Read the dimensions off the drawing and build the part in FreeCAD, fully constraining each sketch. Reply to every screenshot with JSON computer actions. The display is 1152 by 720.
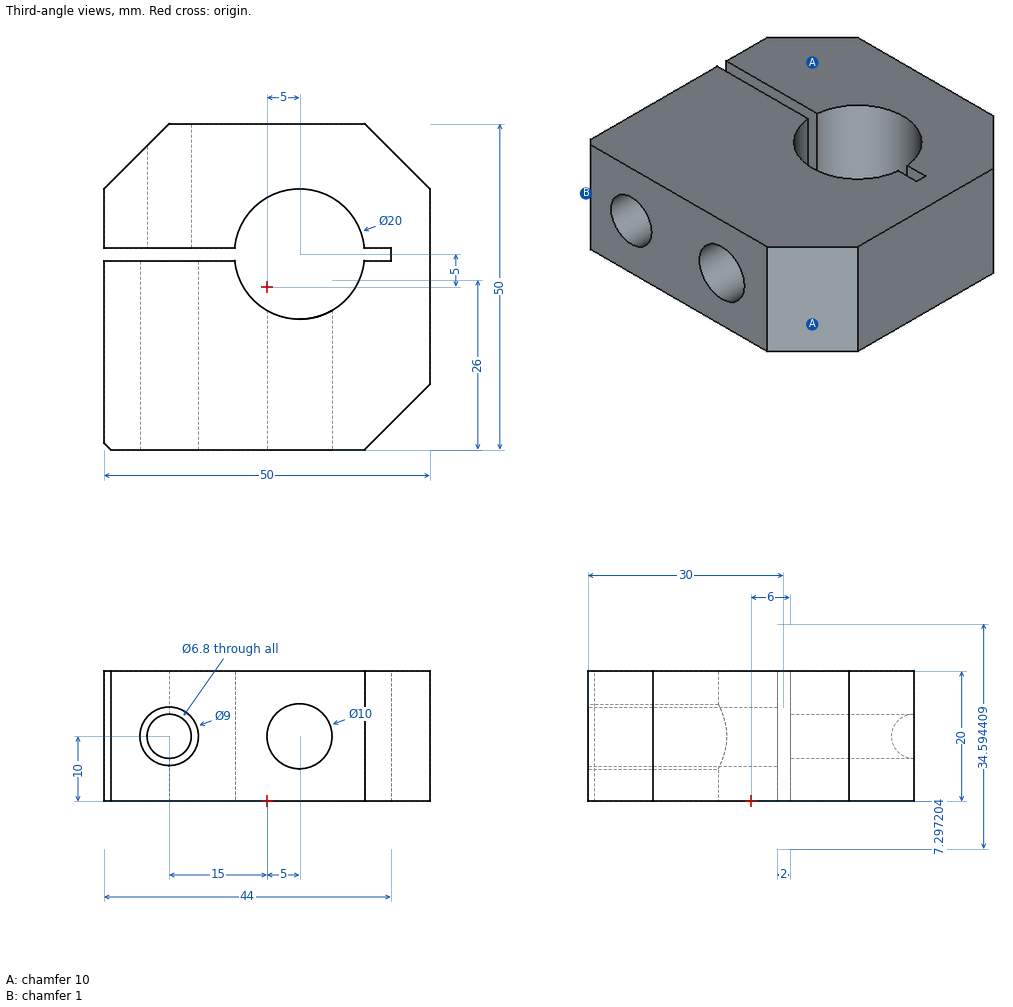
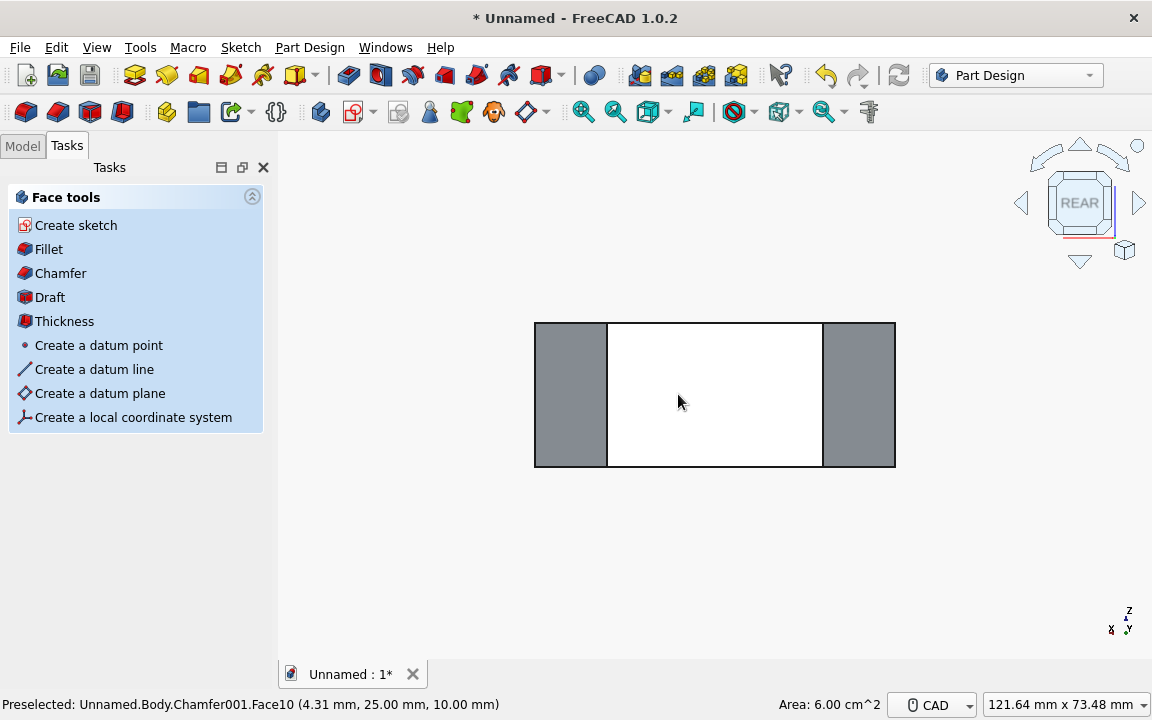
{"action": "left_click", "coordinate": [354, 112]}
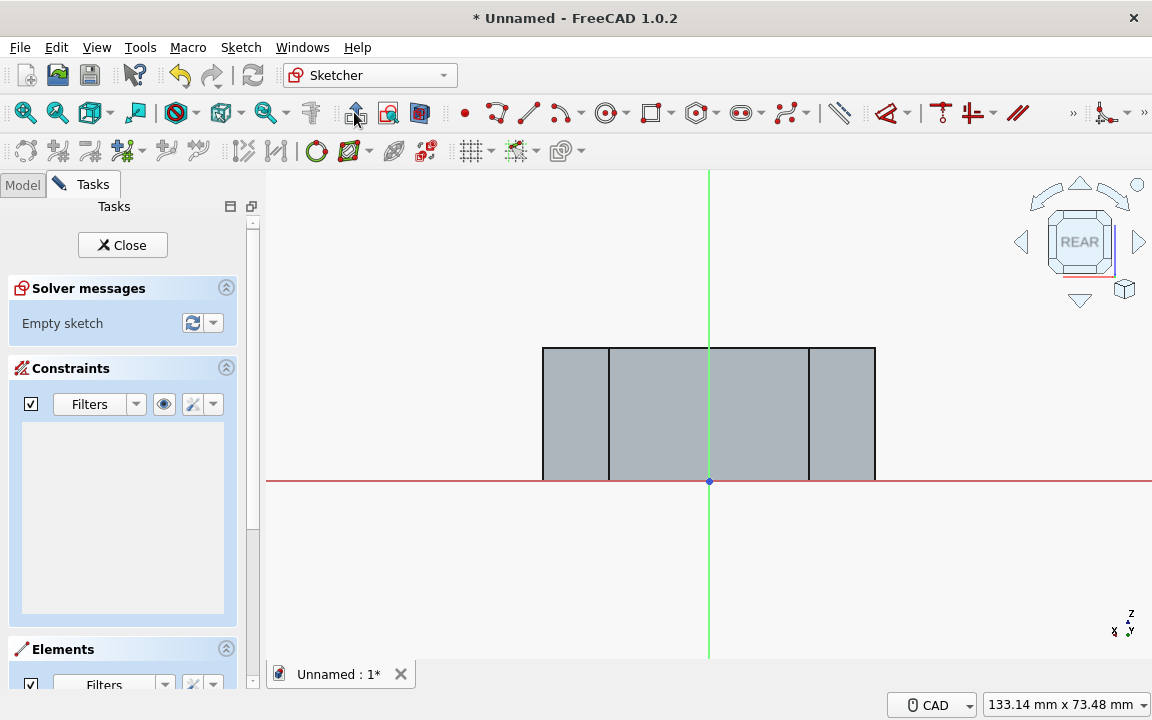
{"action": "scroll", "coordinate": [835, 414], "scroll_direction": "up", "scroll_amount": 10}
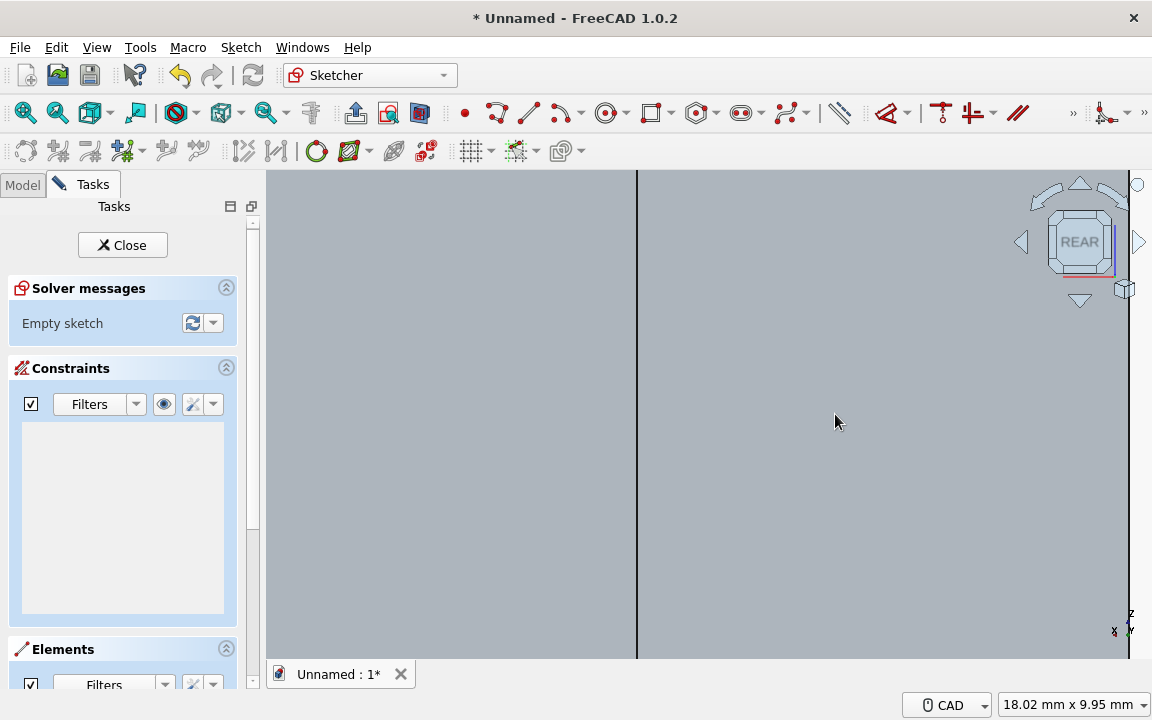
{"action": "left_click", "coordinate": [606, 114]}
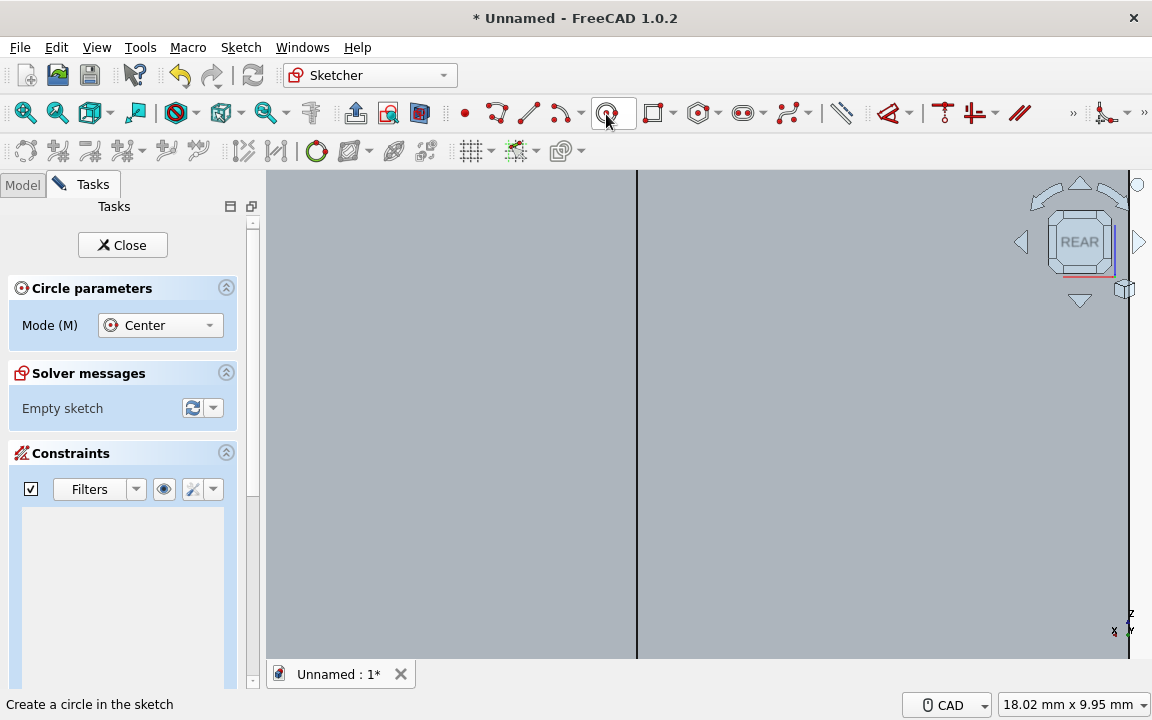
{"action": "left_click", "coordinate": [637, 415]}
{"action": "mouse_move", "coordinate": [756, 296]}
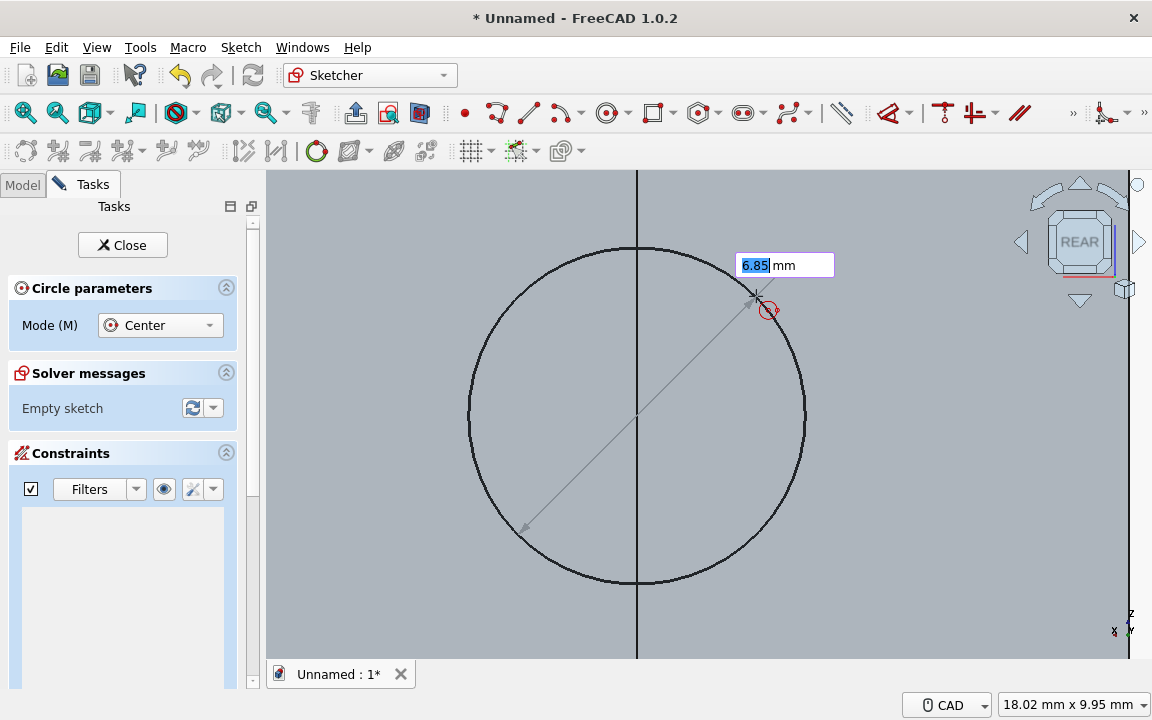
{"action": "type", "text": "6.8"}
{"action": "key", "text": "Return"}
{"action": "key", "text": "Escape"}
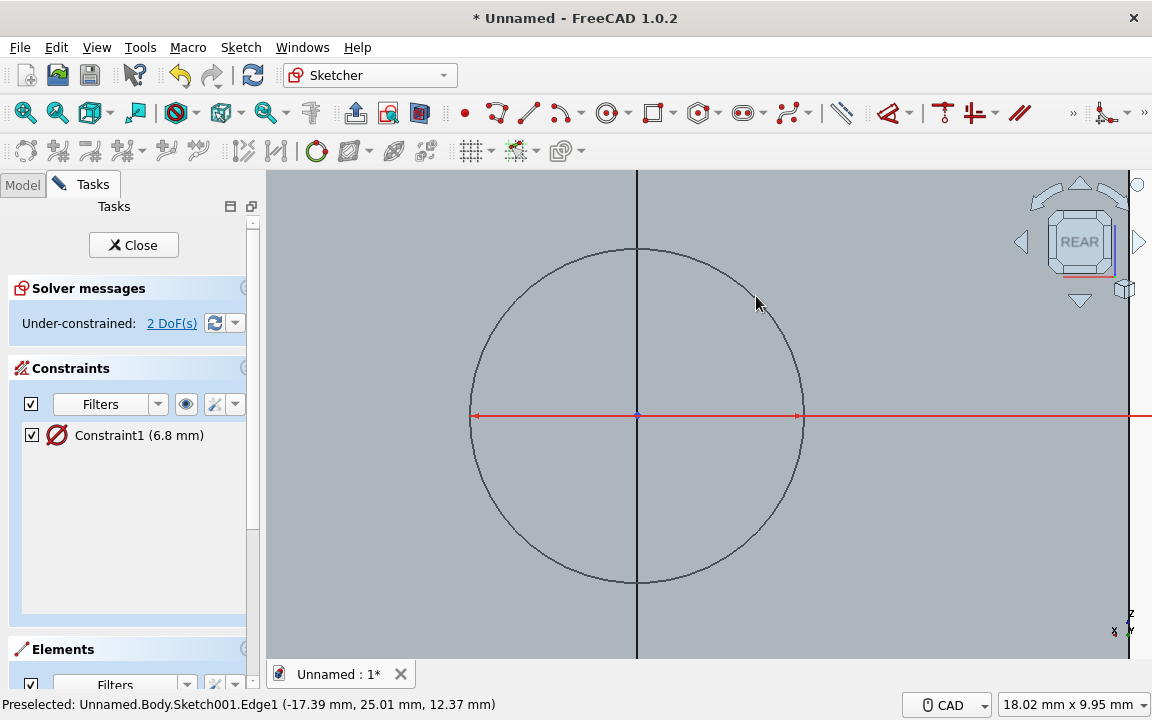
{"action": "left_click", "coordinate": [888, 114]}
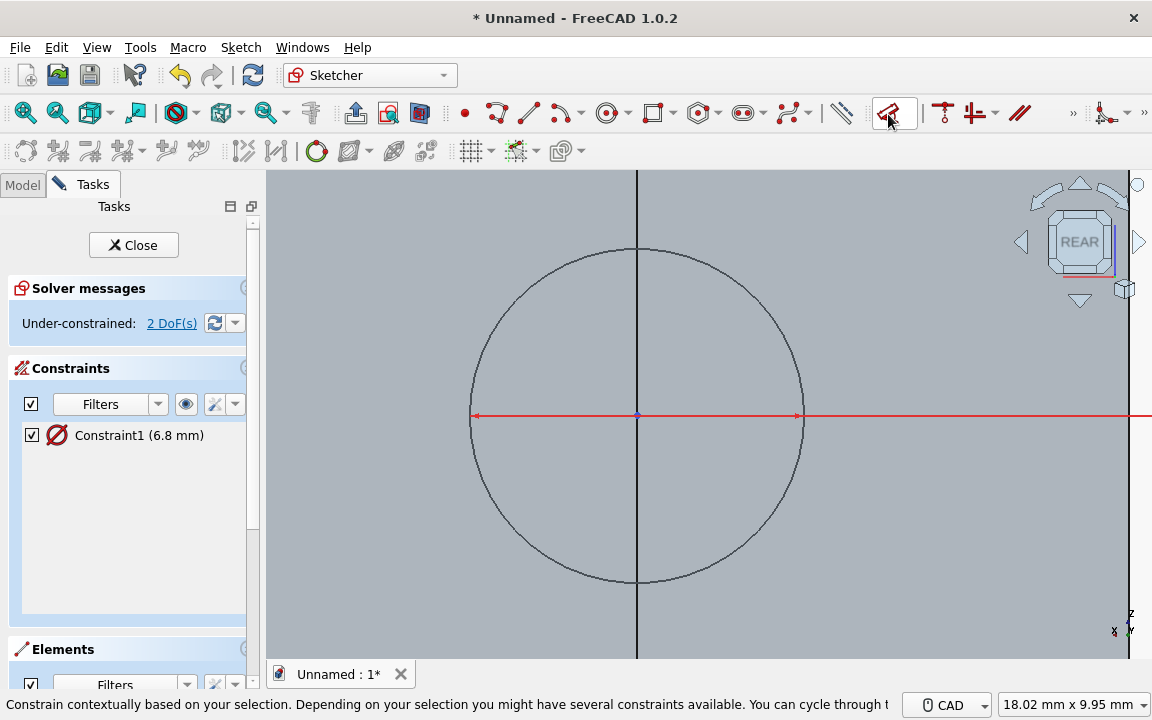
{"action": "left_click", "coordinate": [637, 416]}
{"action": "left_click", "coordinate": [387, 382]}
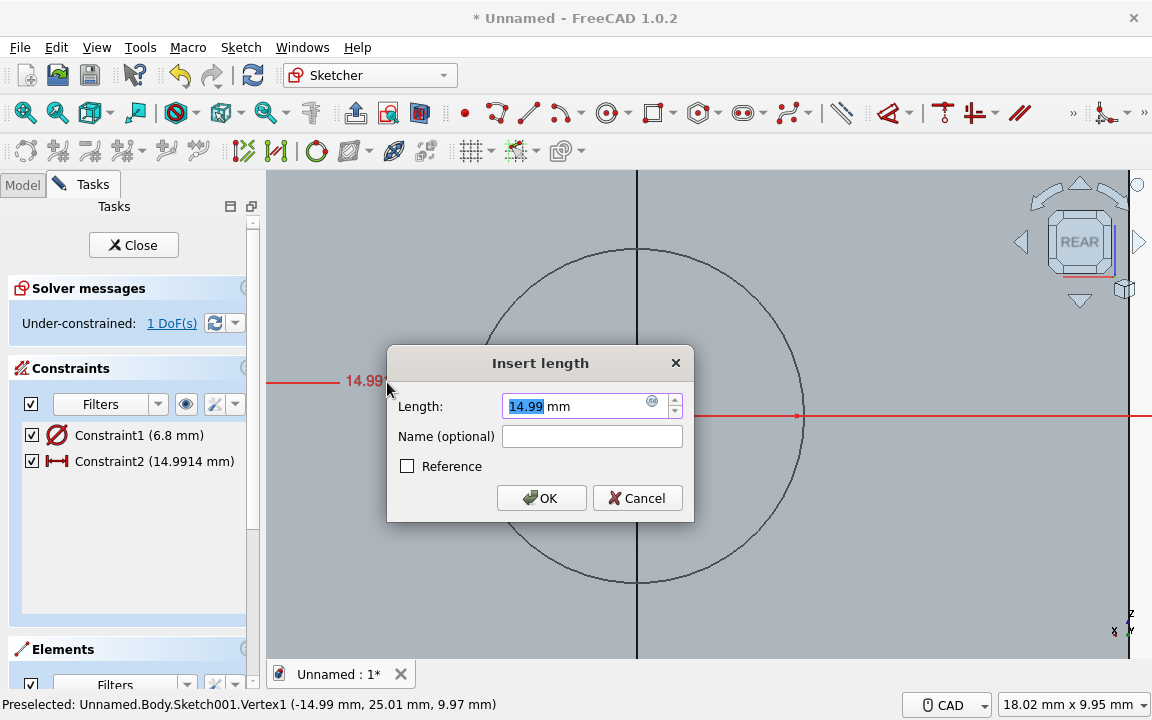
{"action": "type", "text": "15"}
{"action": "key", "text": "Return"}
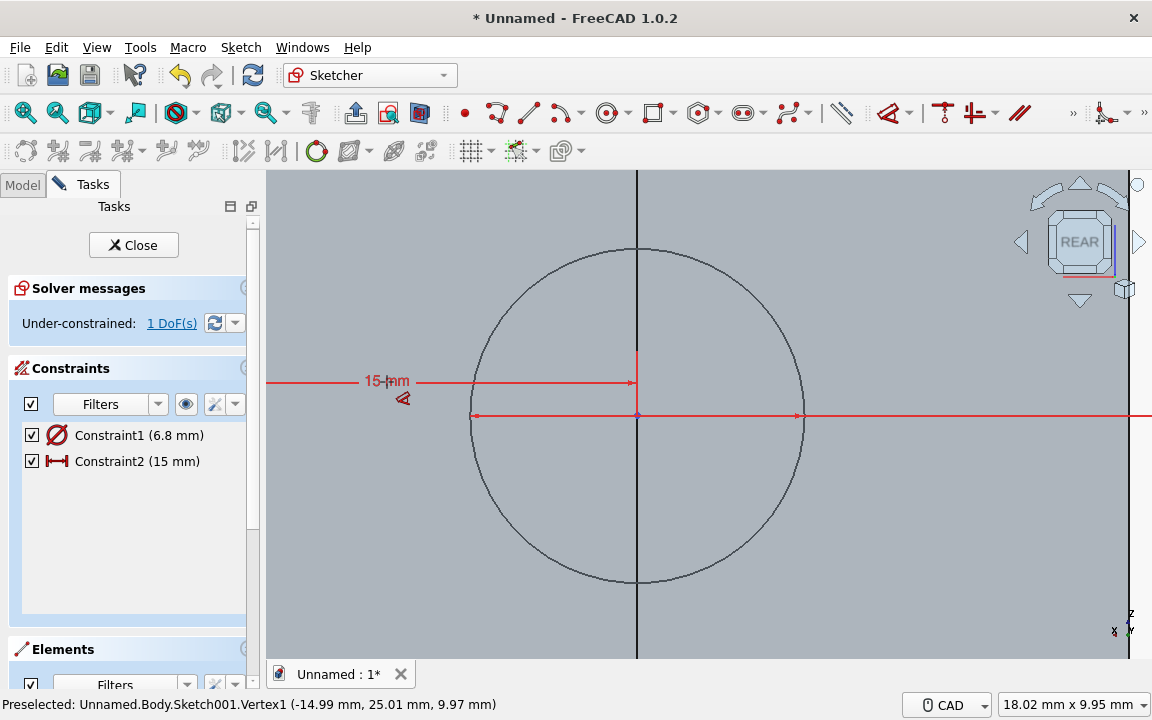
{"action": "left_click", "coordinate": [637, 416]}
{"action": "left_click", "coordinate": [671, 523]}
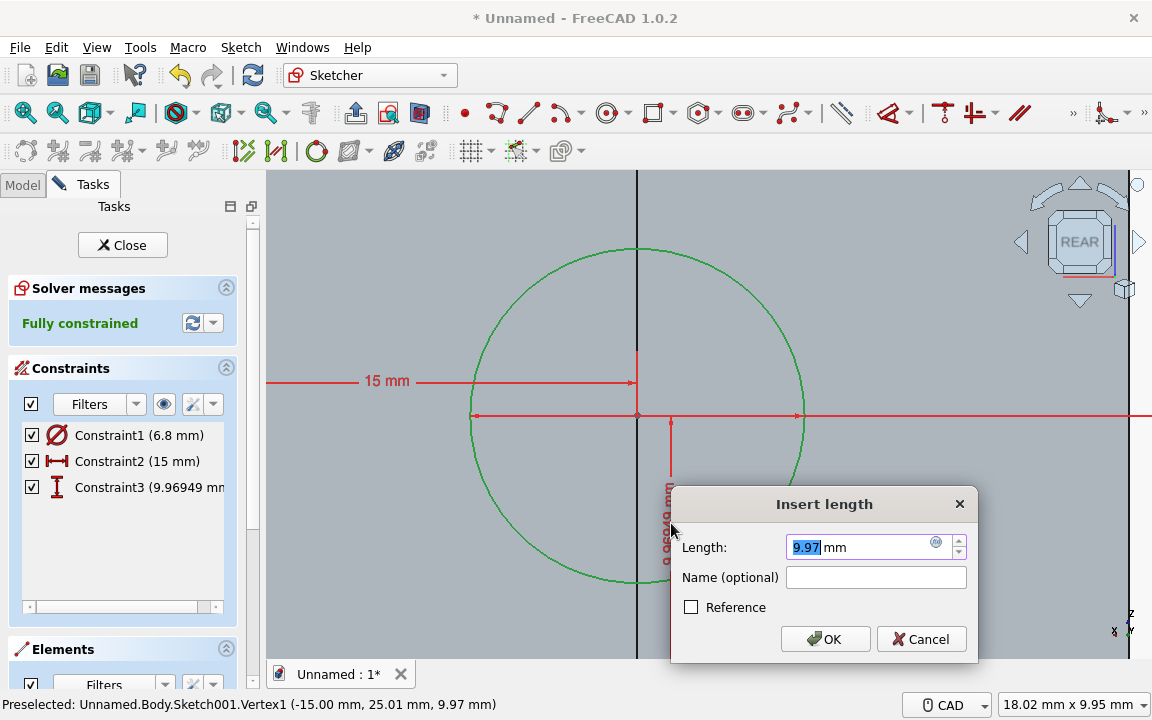
{"action": "type", "text": "10"}
{"action": "key", "text": "Return"}
{"action": "key", "text": "Escape"}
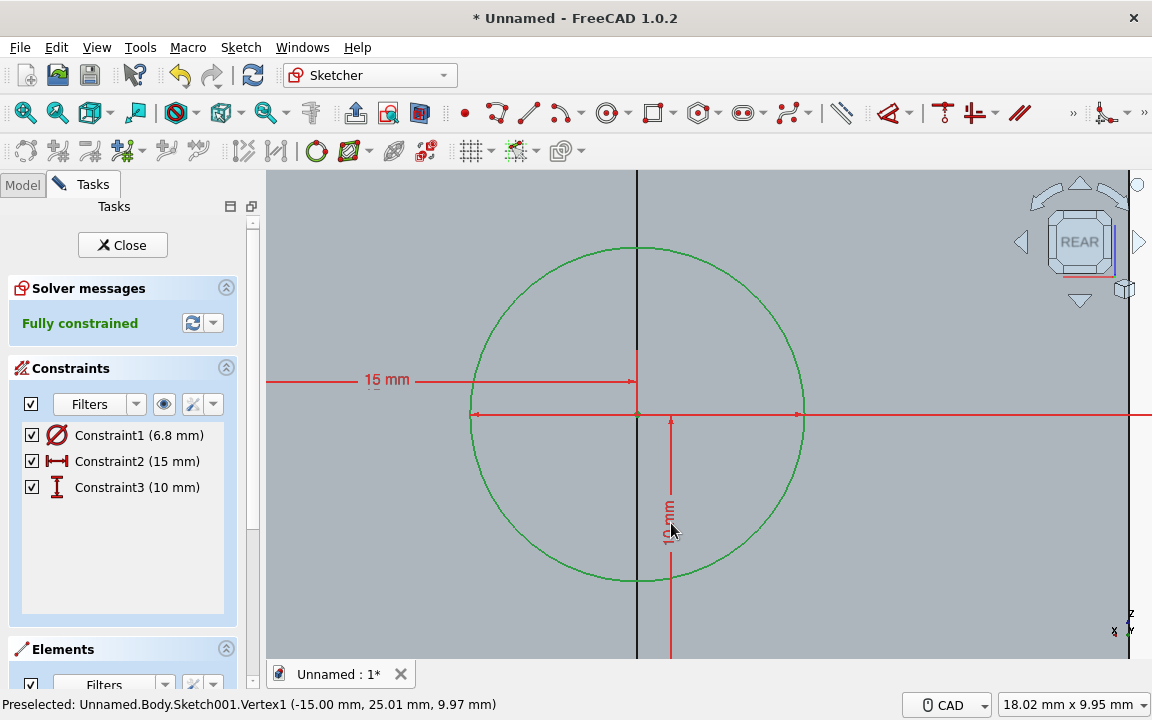
{"action": "left_click", "coordinate": [123, 245]}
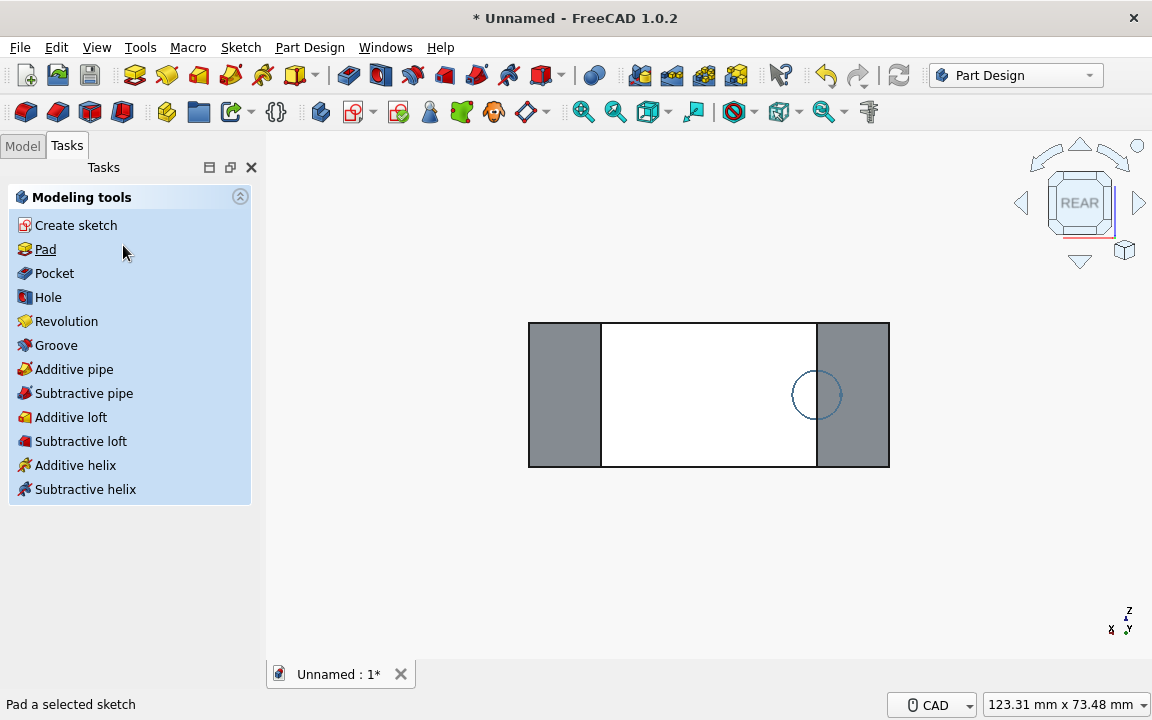
{"action": "left_click", "coordinate": [382, 76]}